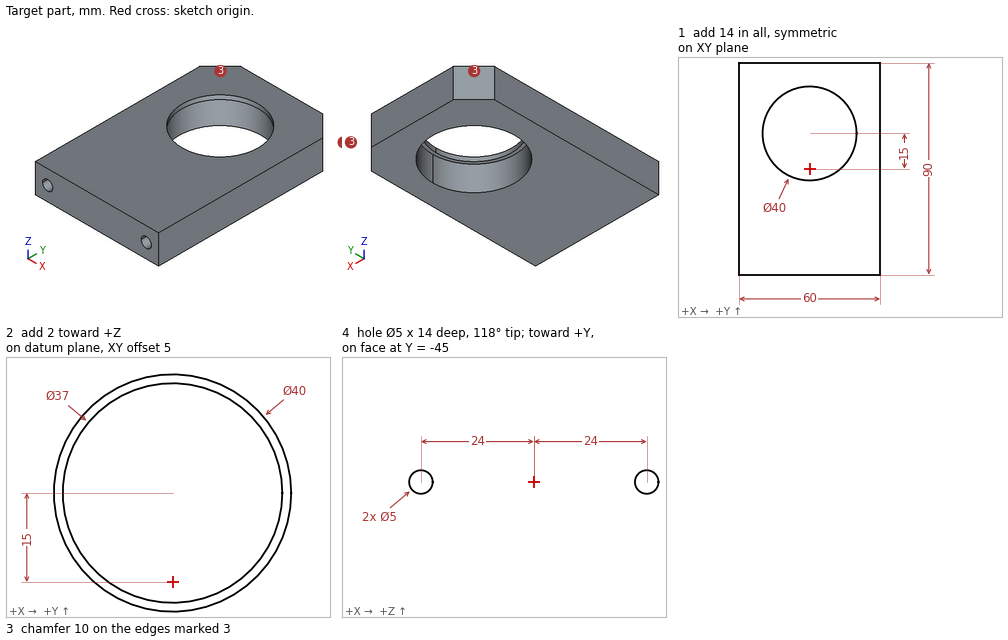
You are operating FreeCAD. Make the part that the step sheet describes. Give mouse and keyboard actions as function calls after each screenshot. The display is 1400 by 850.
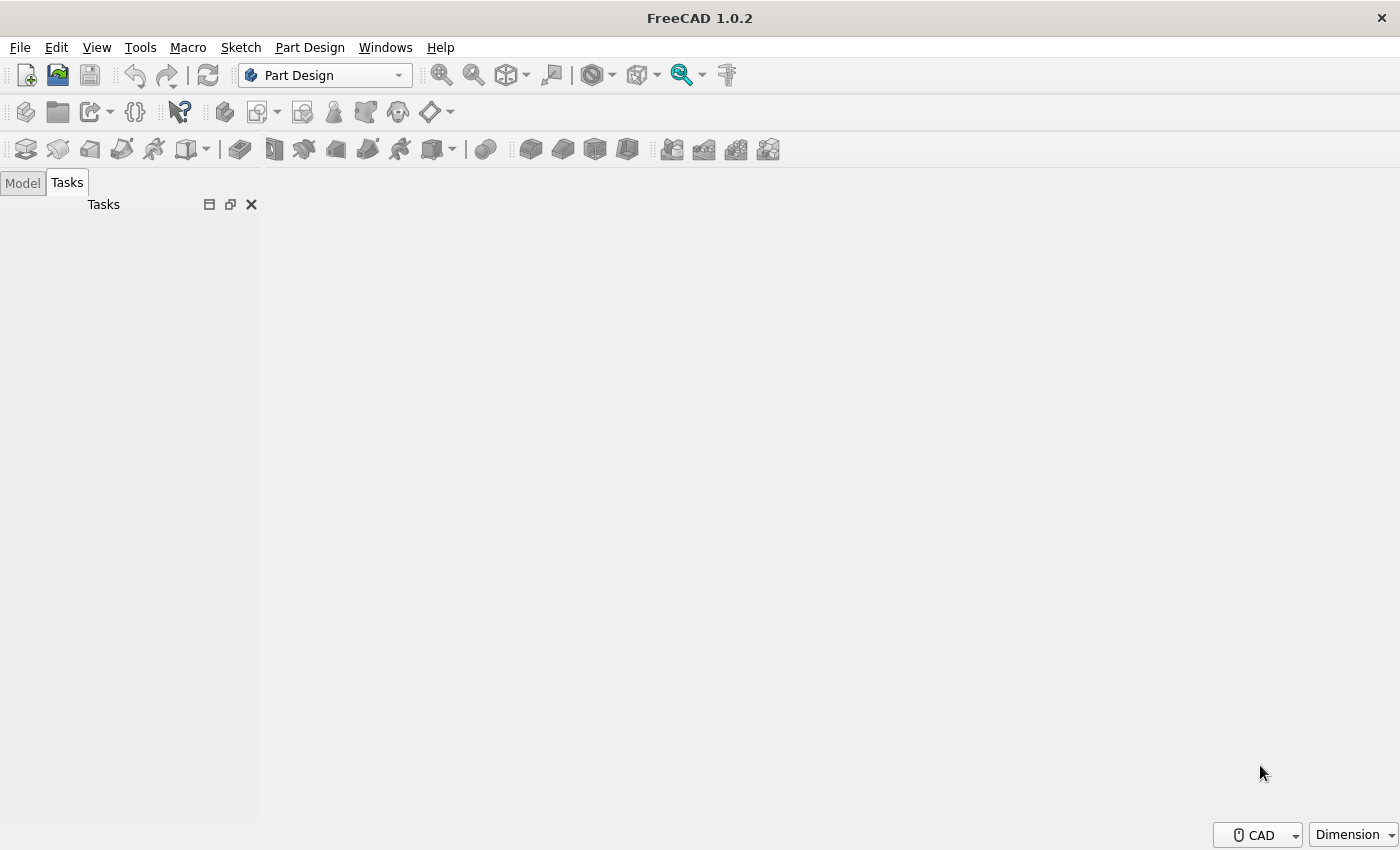
click(980, 76)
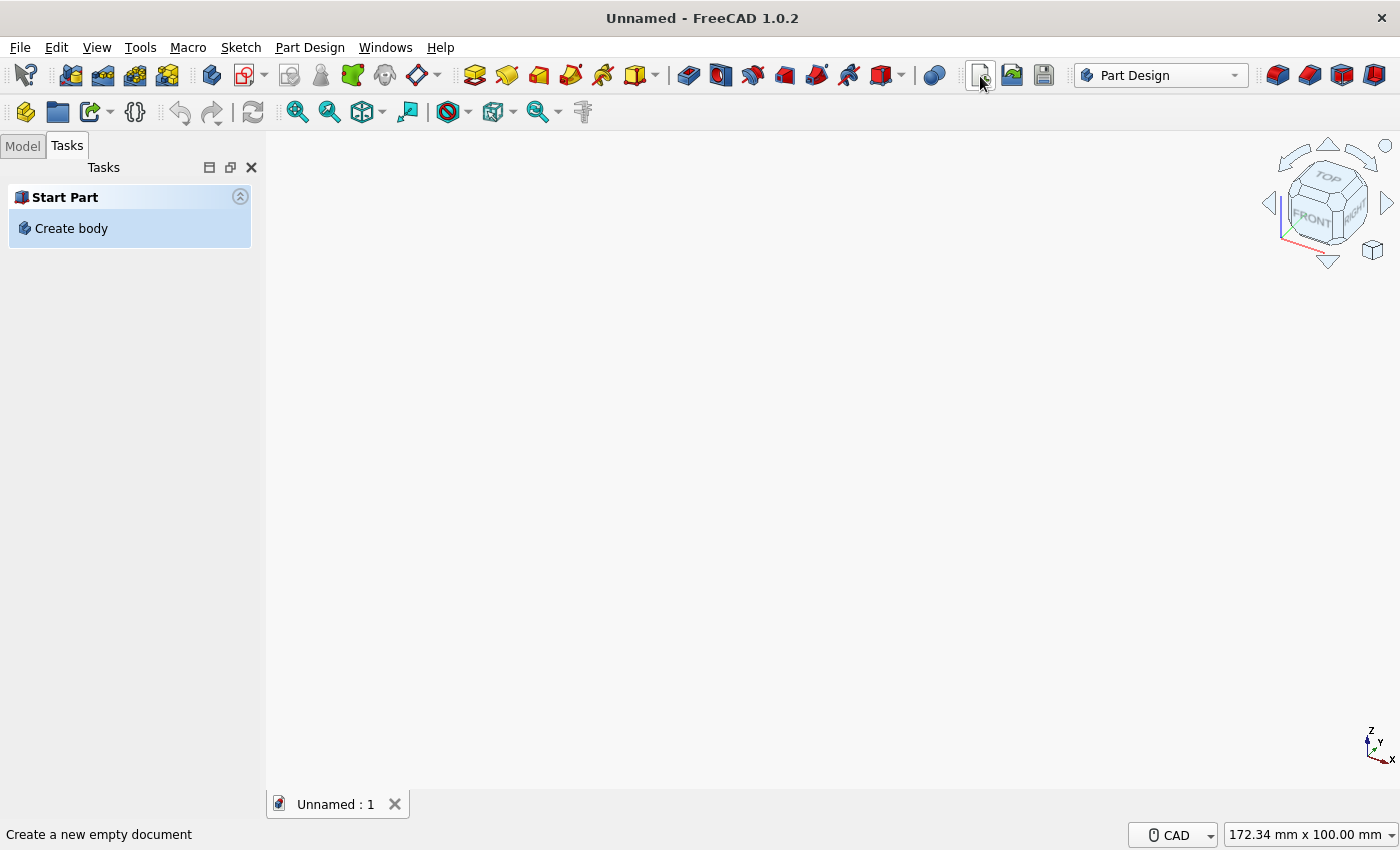
click(244, 76)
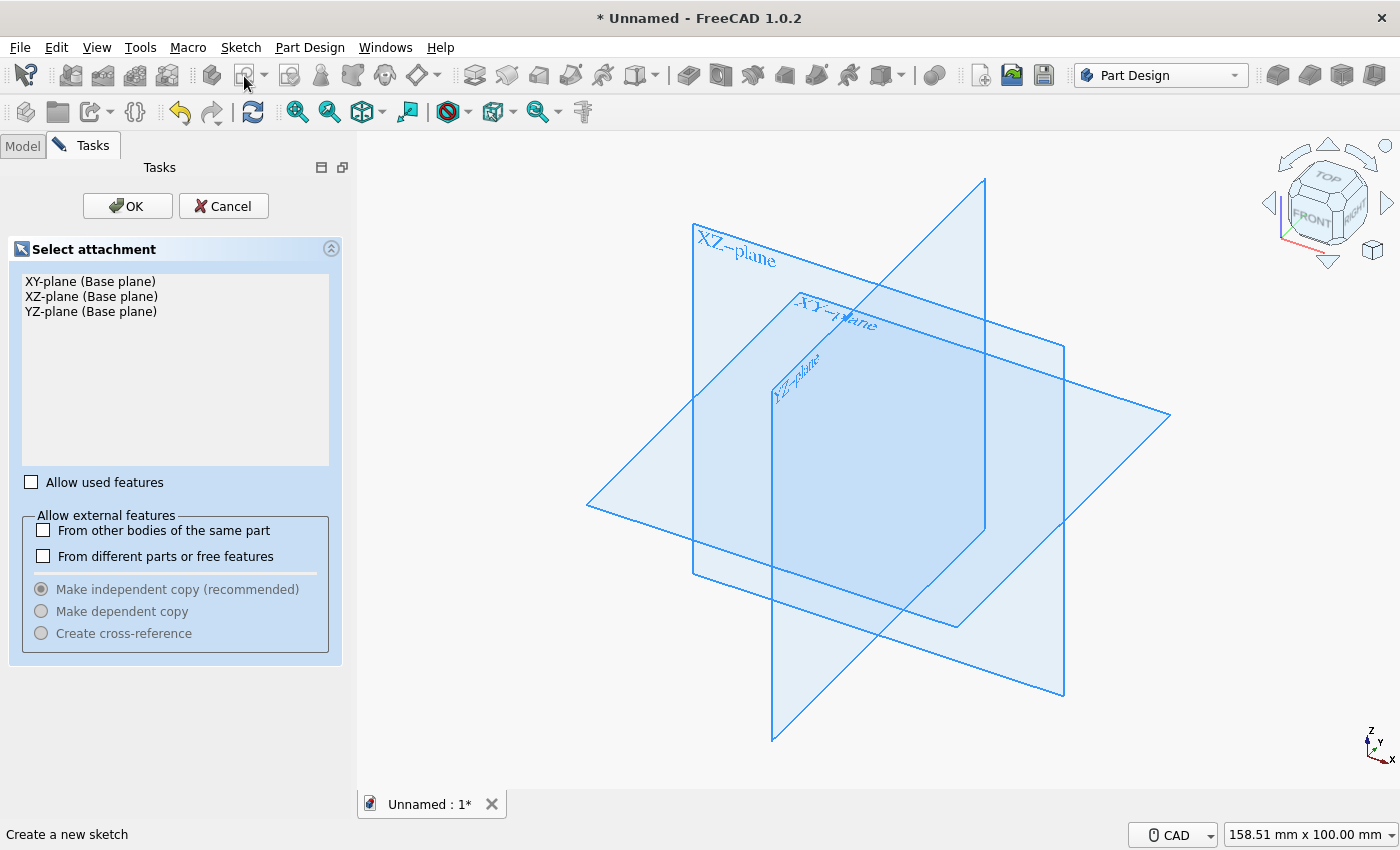
click(82, 282)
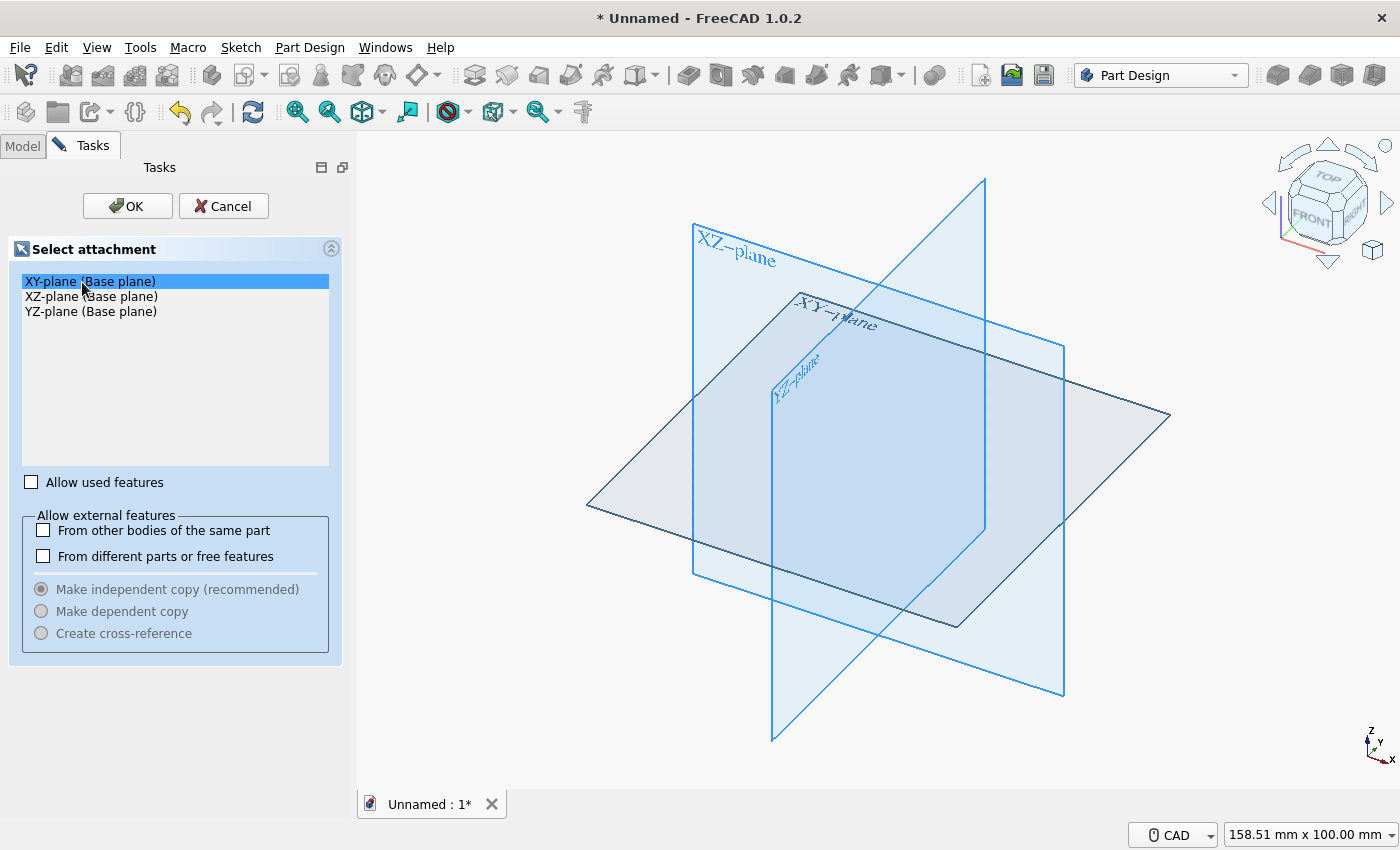
click(128, 206)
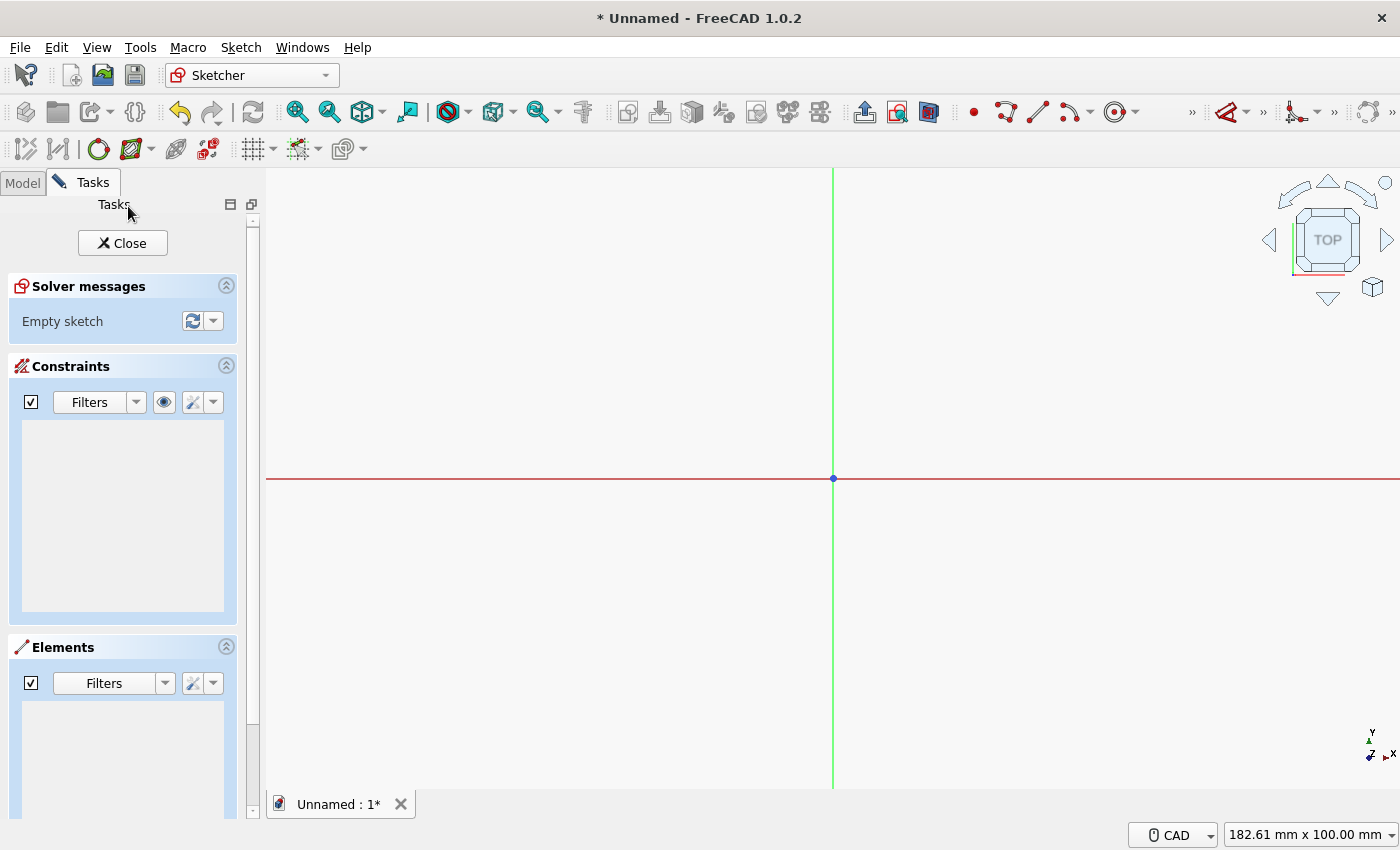
scroll(625, 479, down, 2)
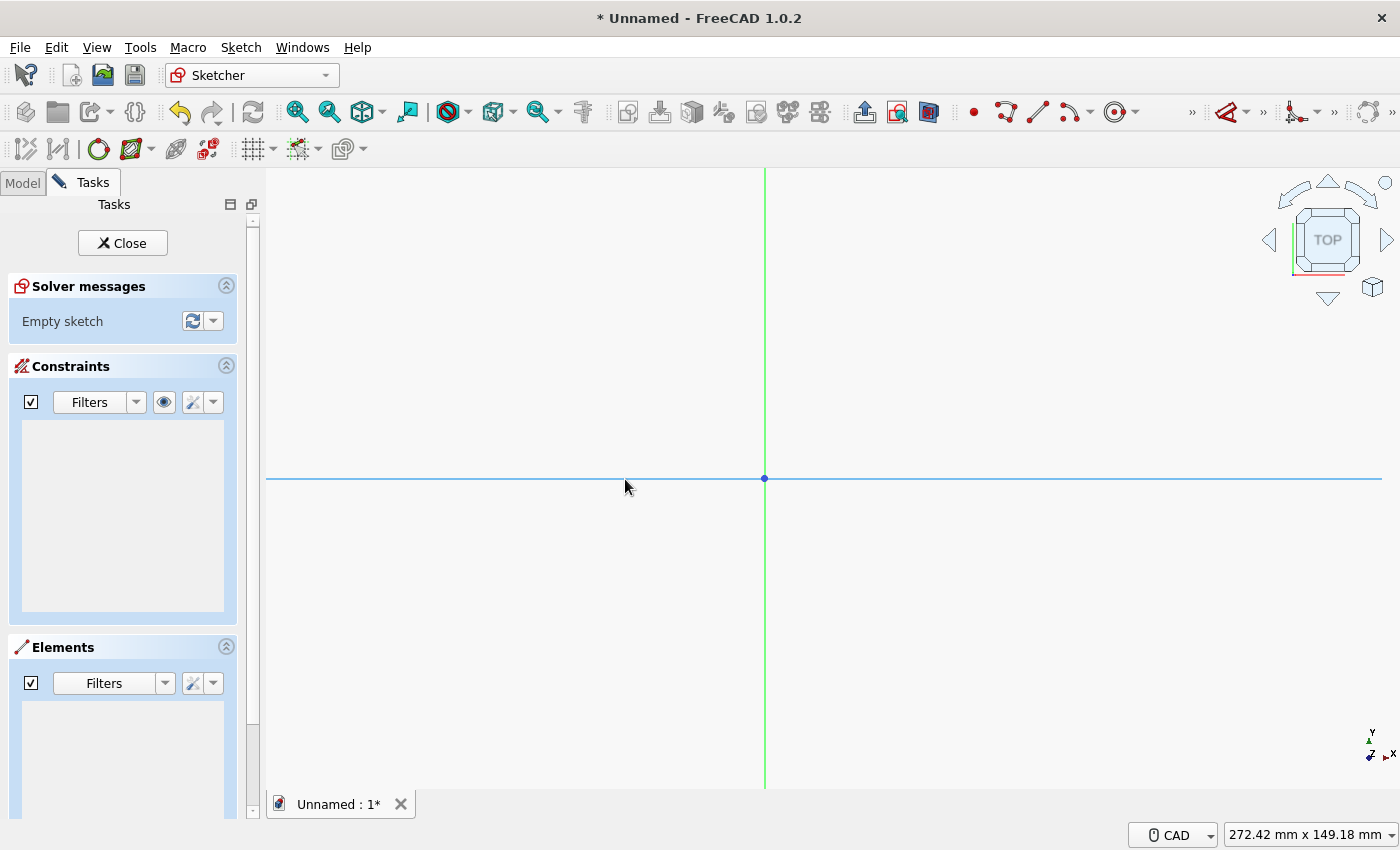
key(g)
key(v)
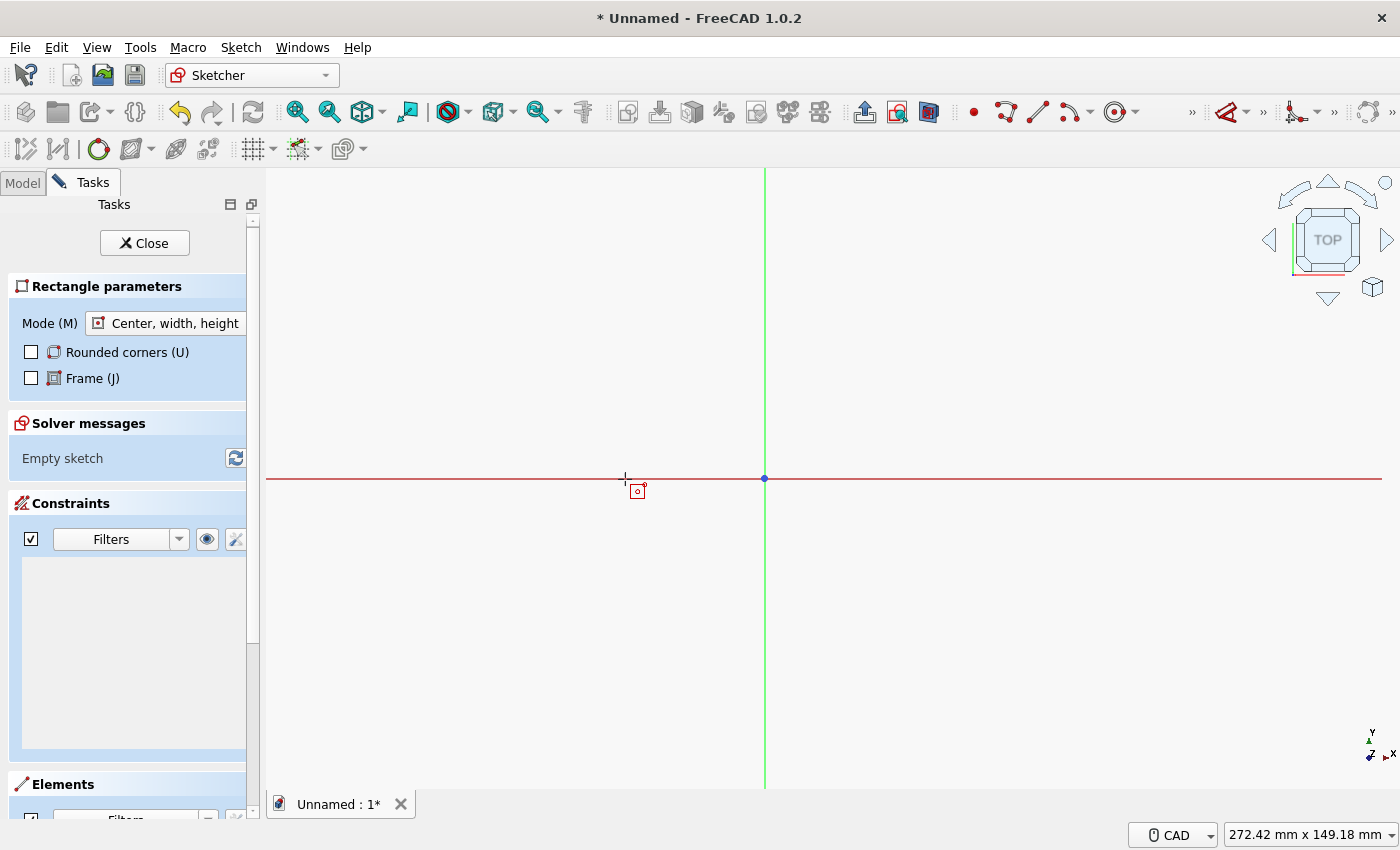
click(765, 479)
move(889, 292)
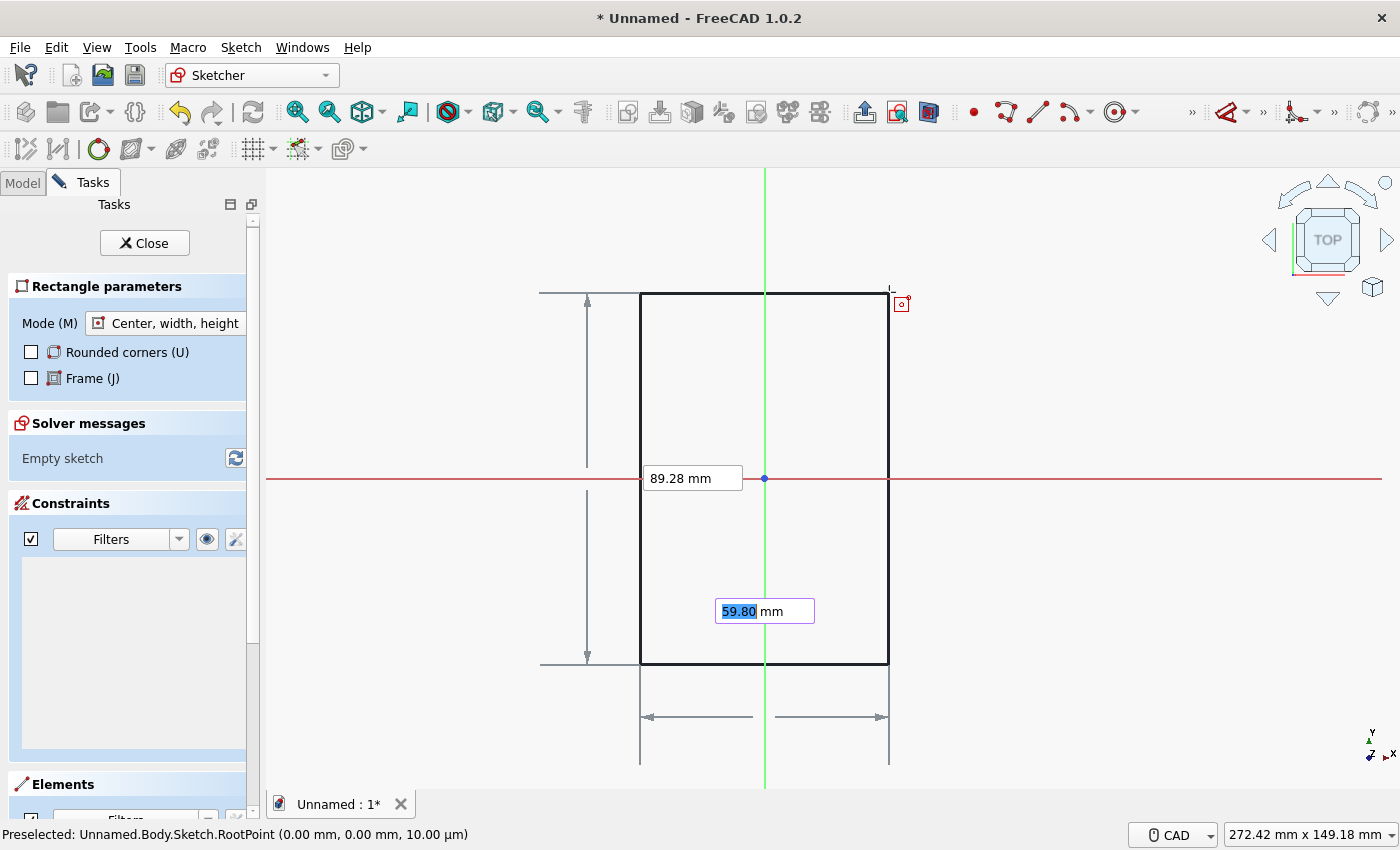
text(60)
key(Tab)
text(90)
key(Return)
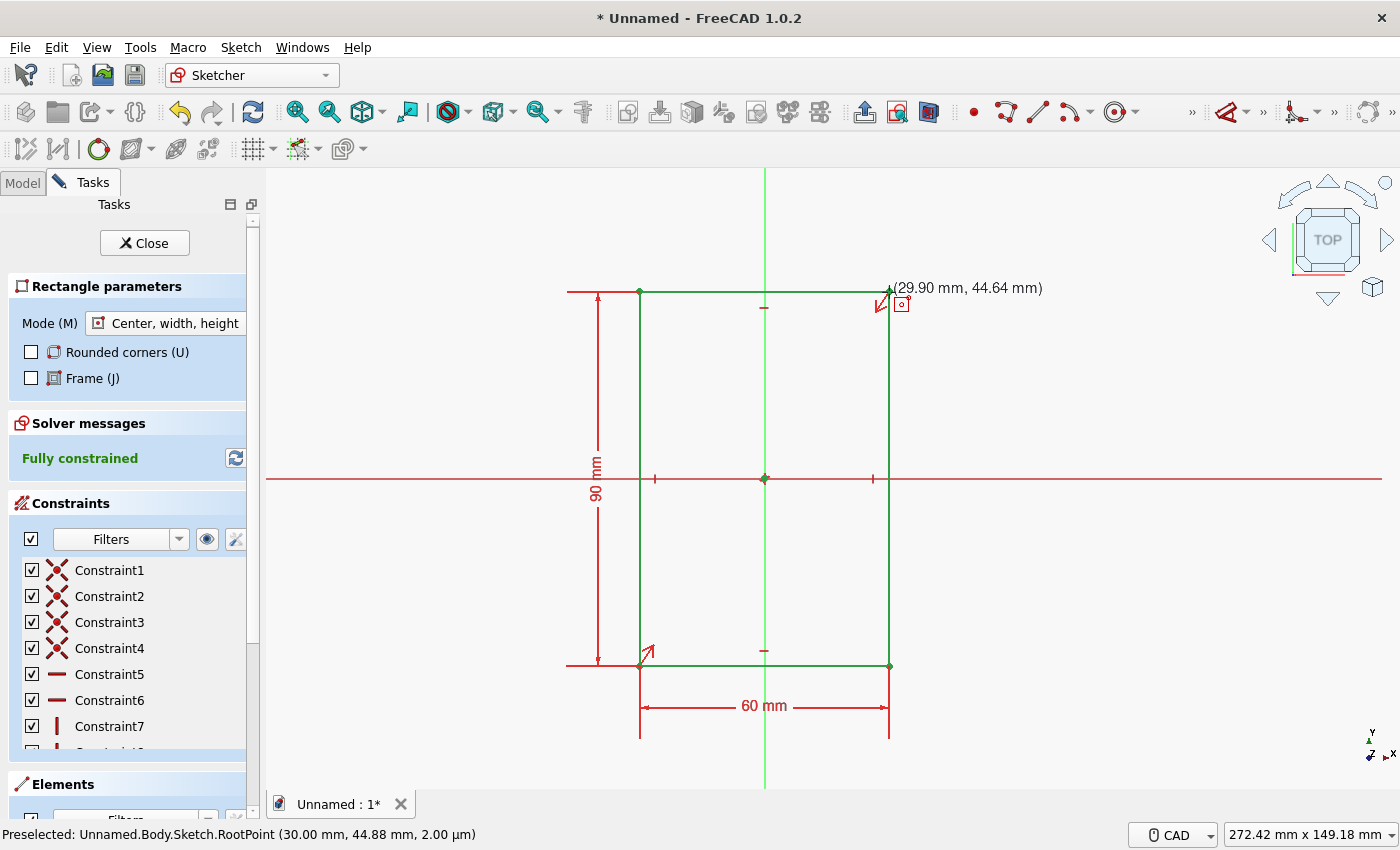
click(1116, 112)